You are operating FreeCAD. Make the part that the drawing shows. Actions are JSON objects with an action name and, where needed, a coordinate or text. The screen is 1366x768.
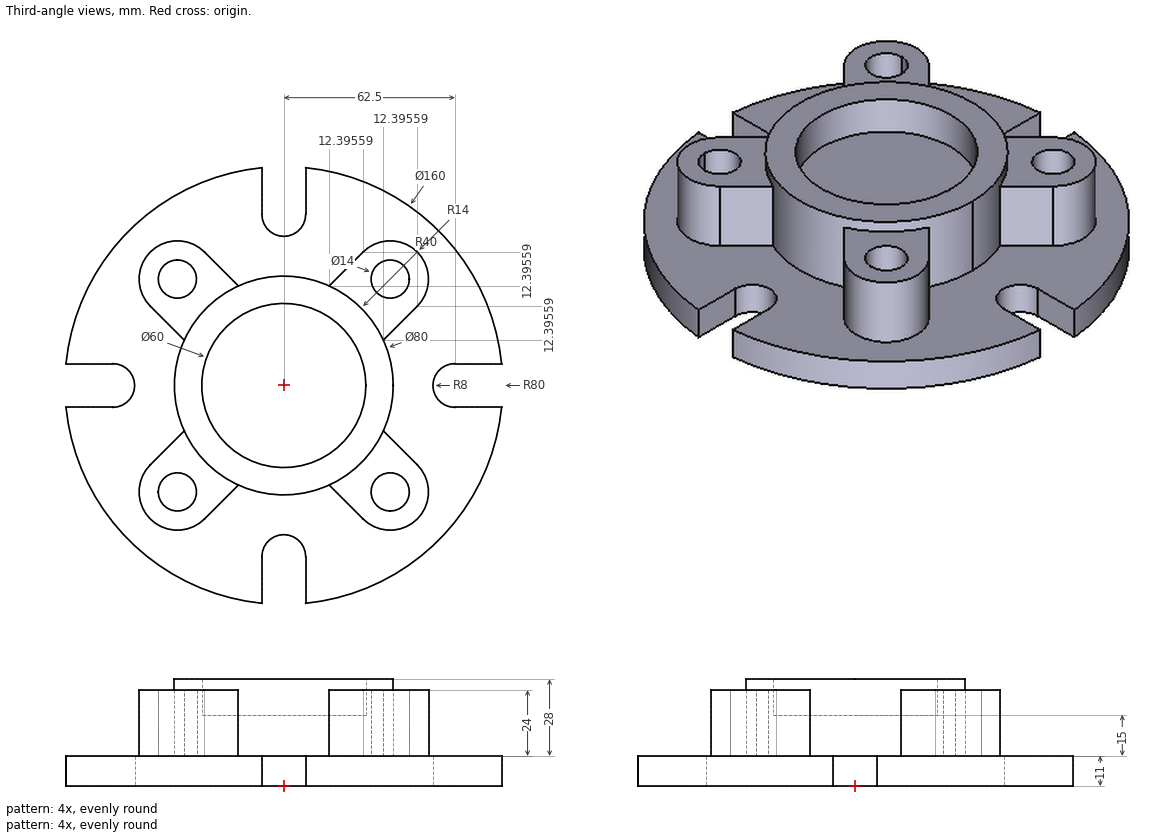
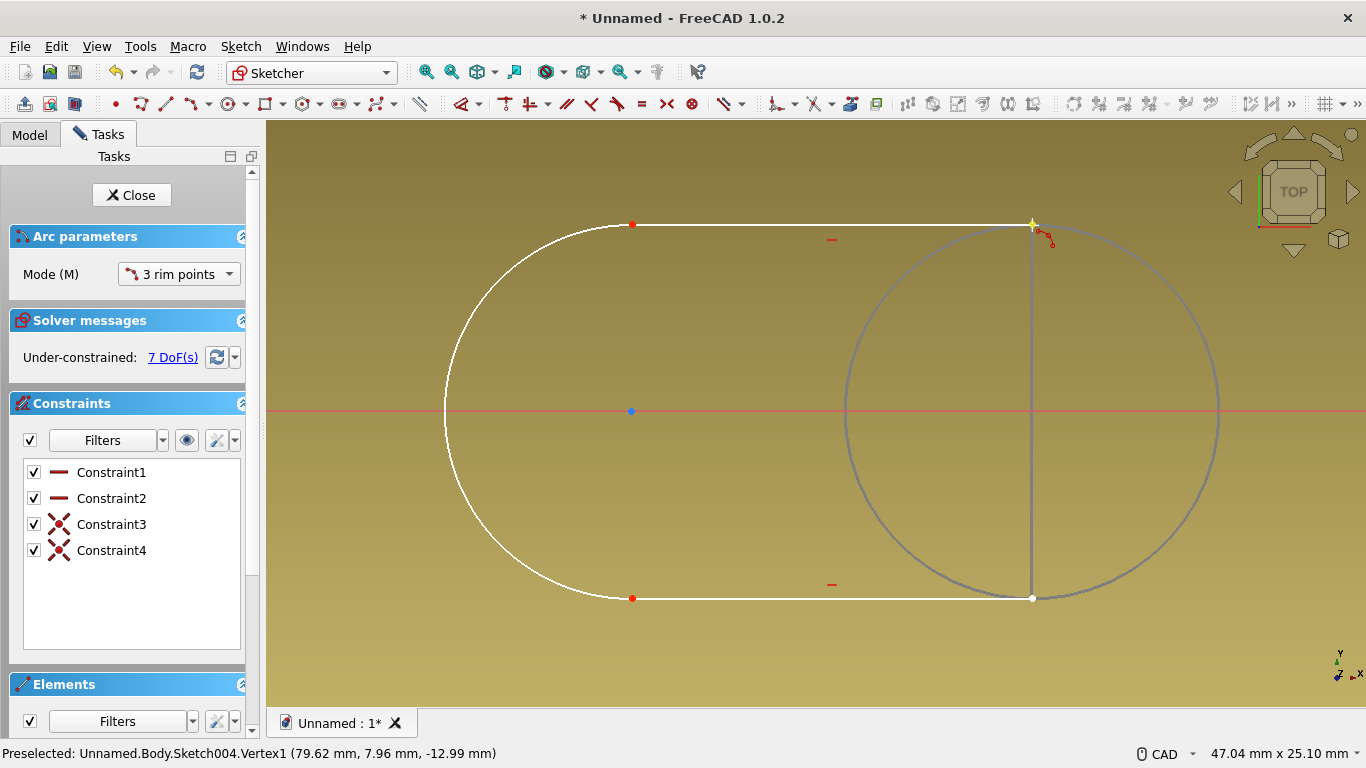
{"action": "scroll", "coordinate": [1041, 449], "scroll_direction": "up", "scroll_amount": 3}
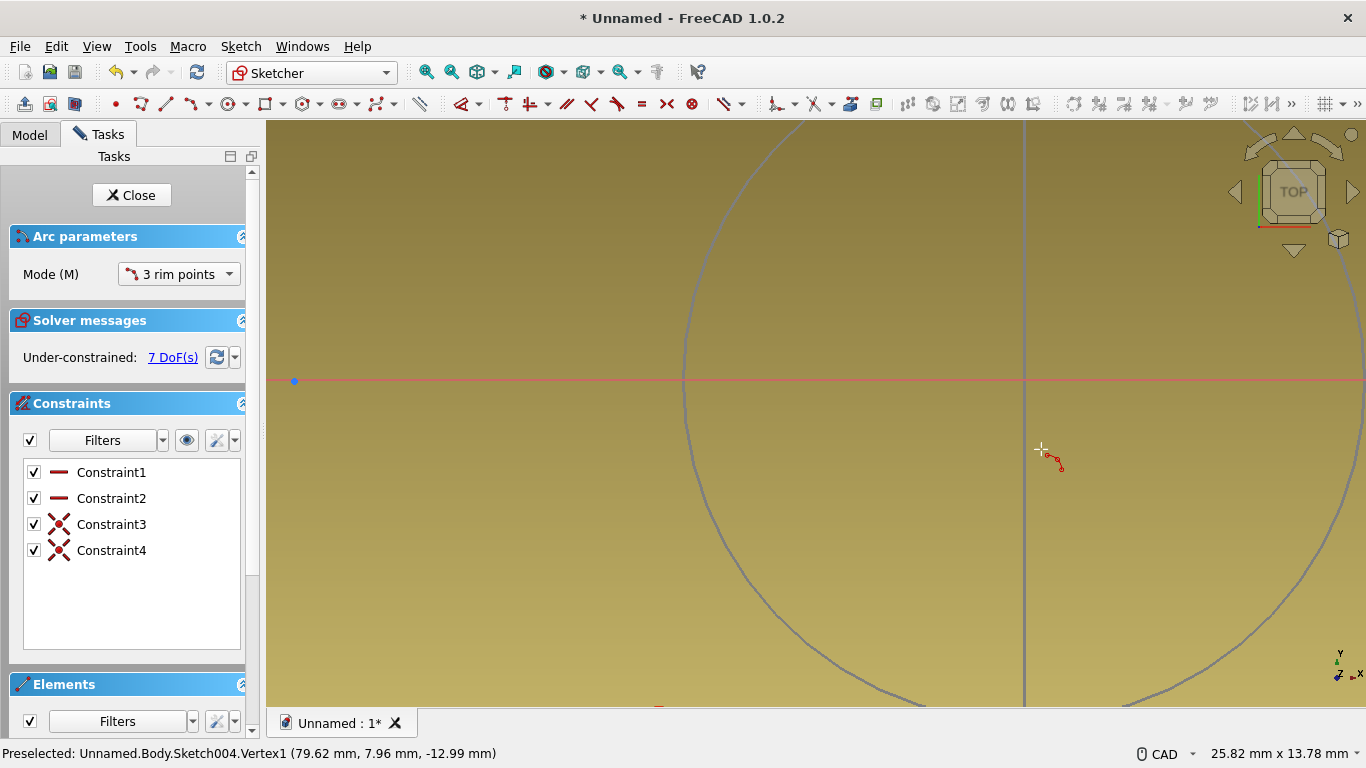
{"action": "left_click", "coordinate": [1040, 448]}
{"action": "key", "text": "Escape"}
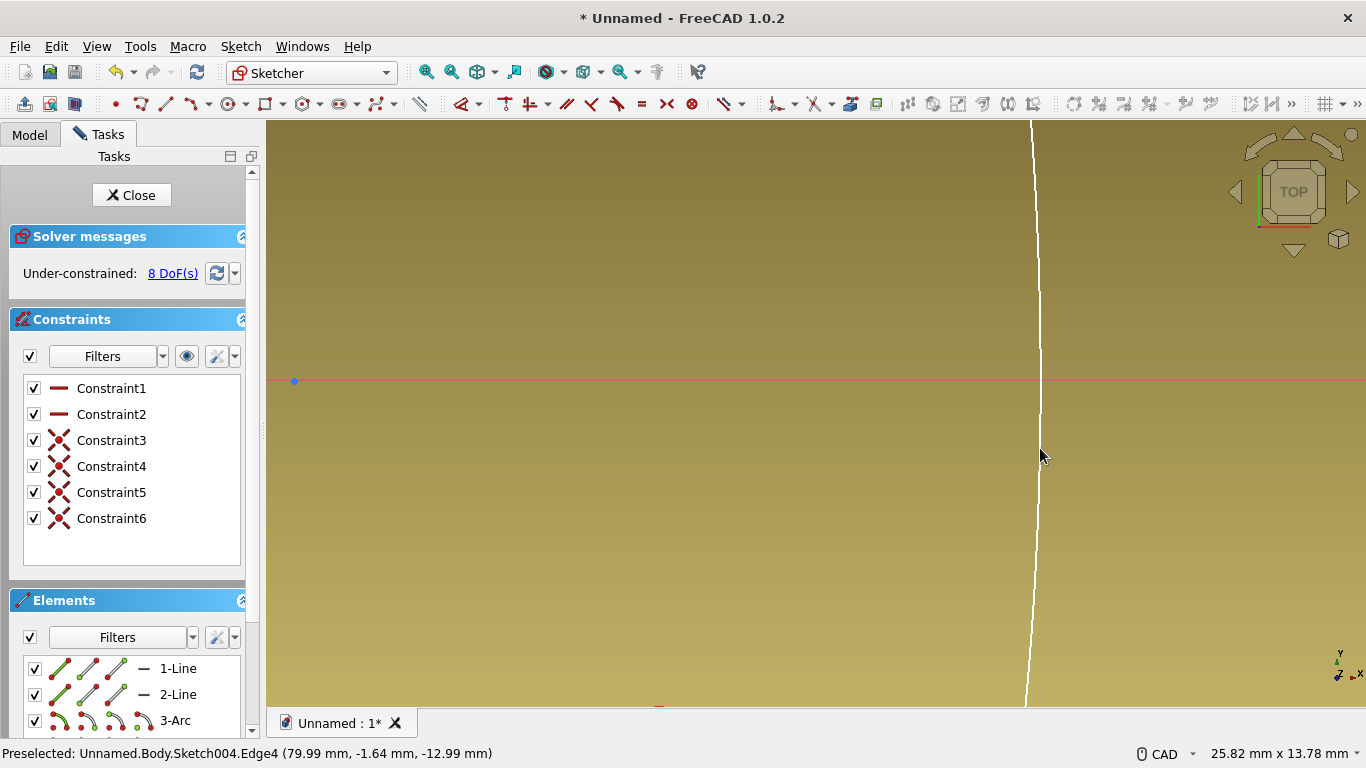
{"action": "scroll", "coordinate": [1052, 455], "scroll_direction": "down", "scroll_amount": 3}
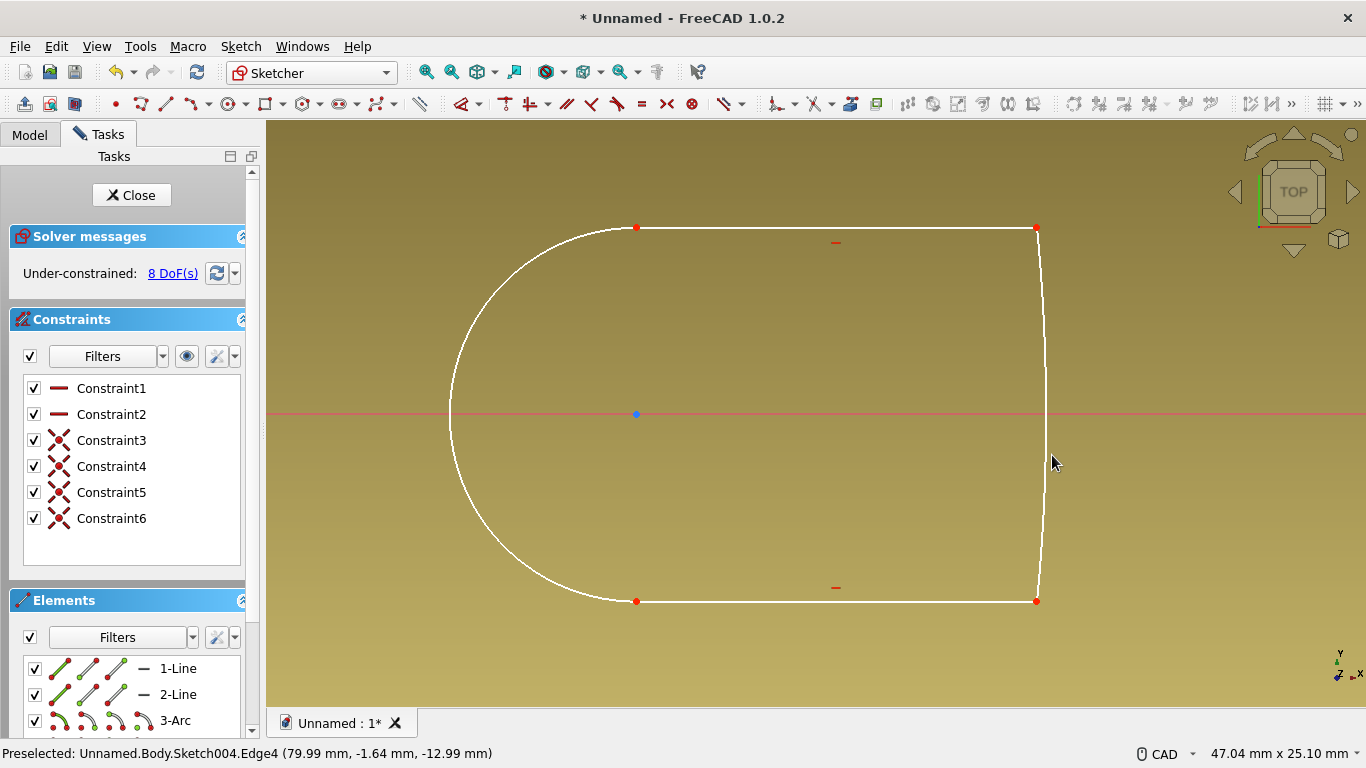
{"action": "left_click", "coordinate": [917, 228]}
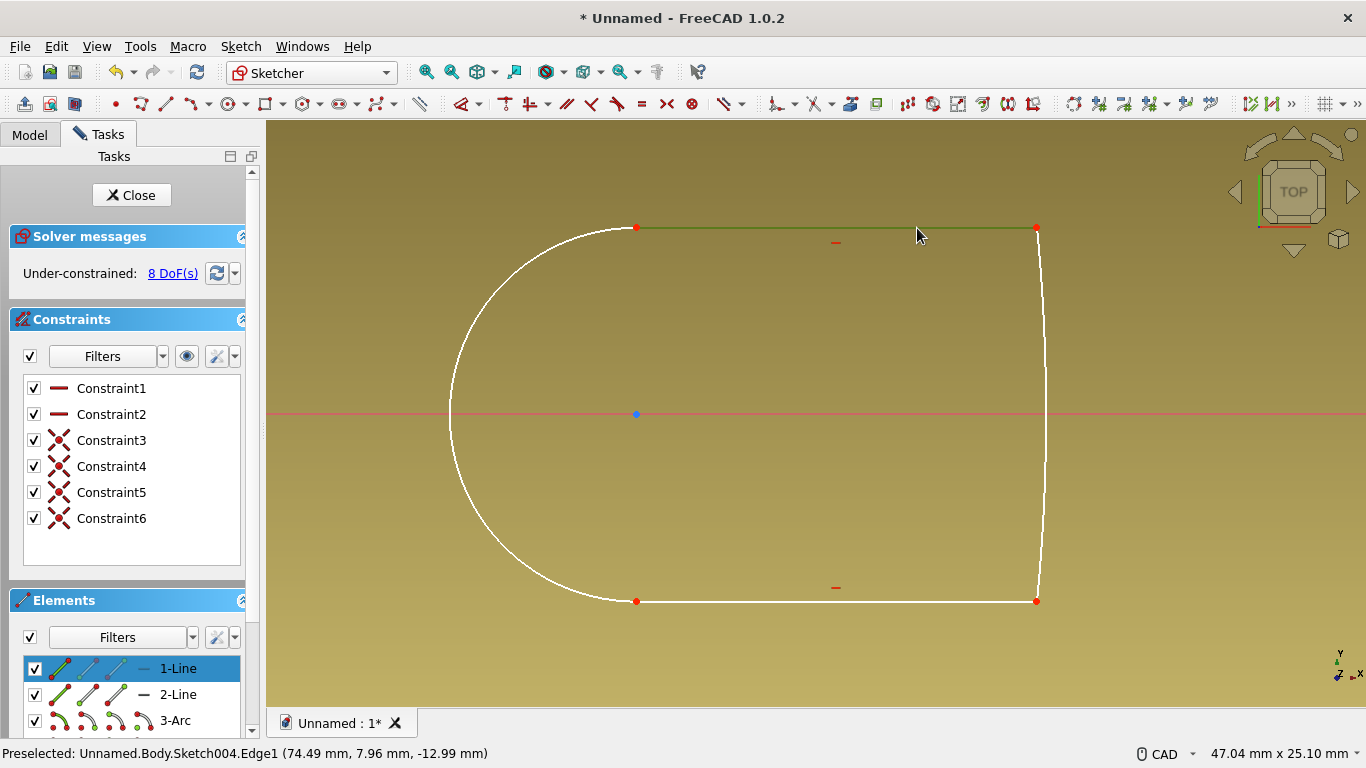
{"action": "left_click", "coordinate": [486, 305]}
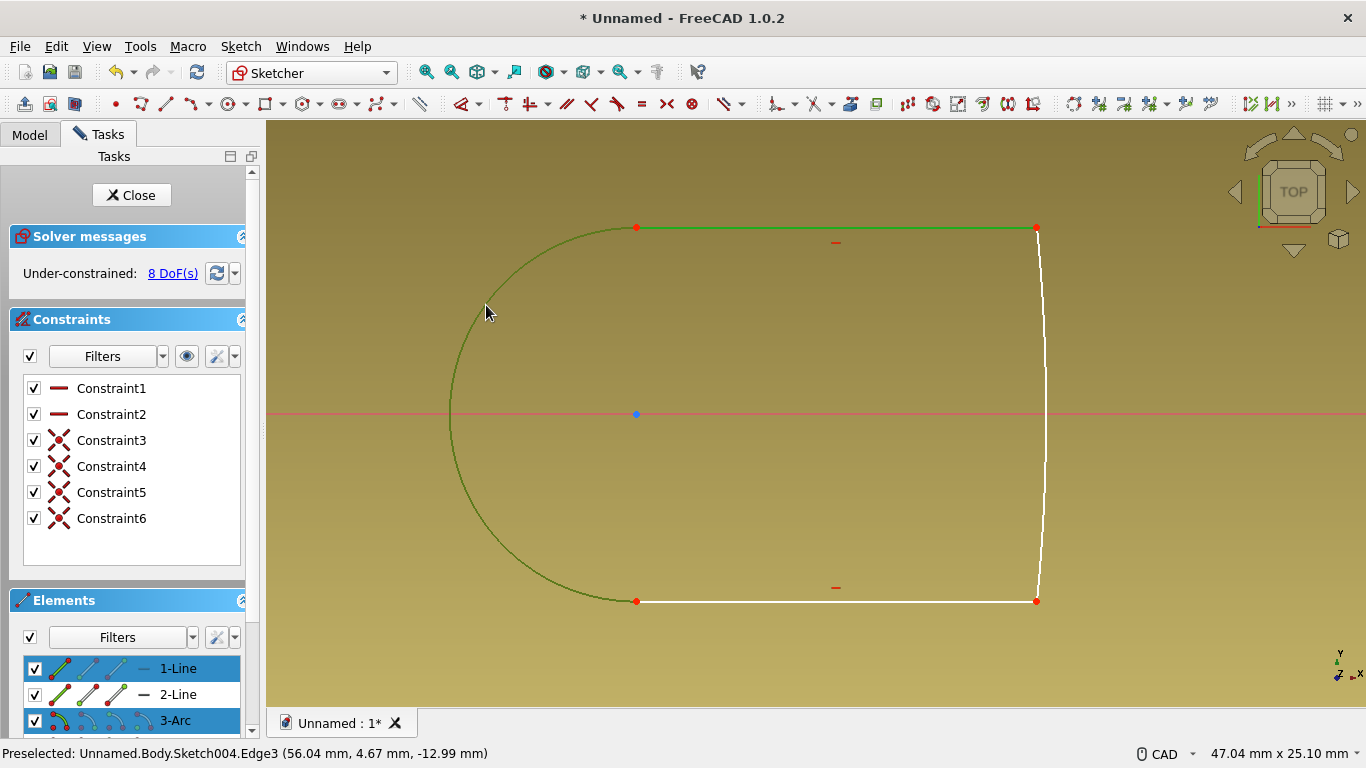
{"action": "key", "text": "t"}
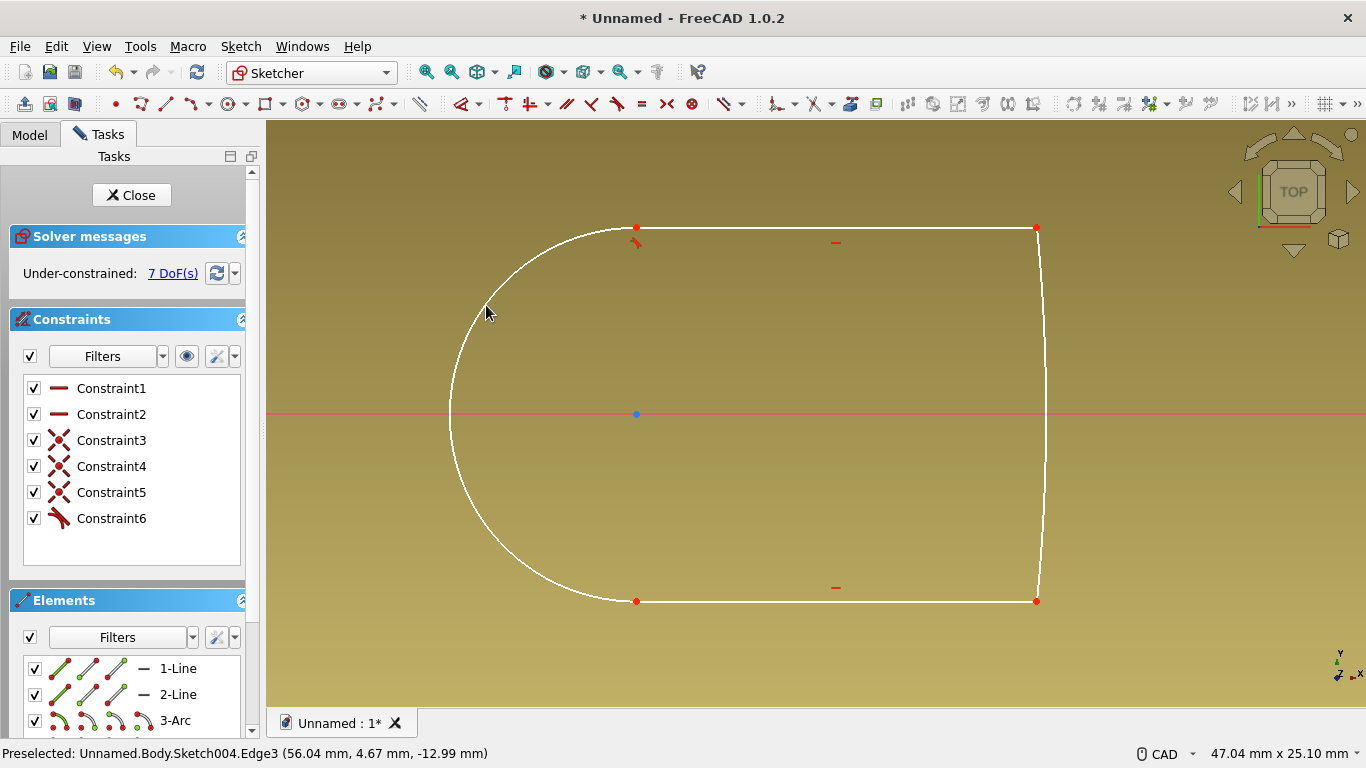
{"action": "left_click", "coordinate": [757, 602]}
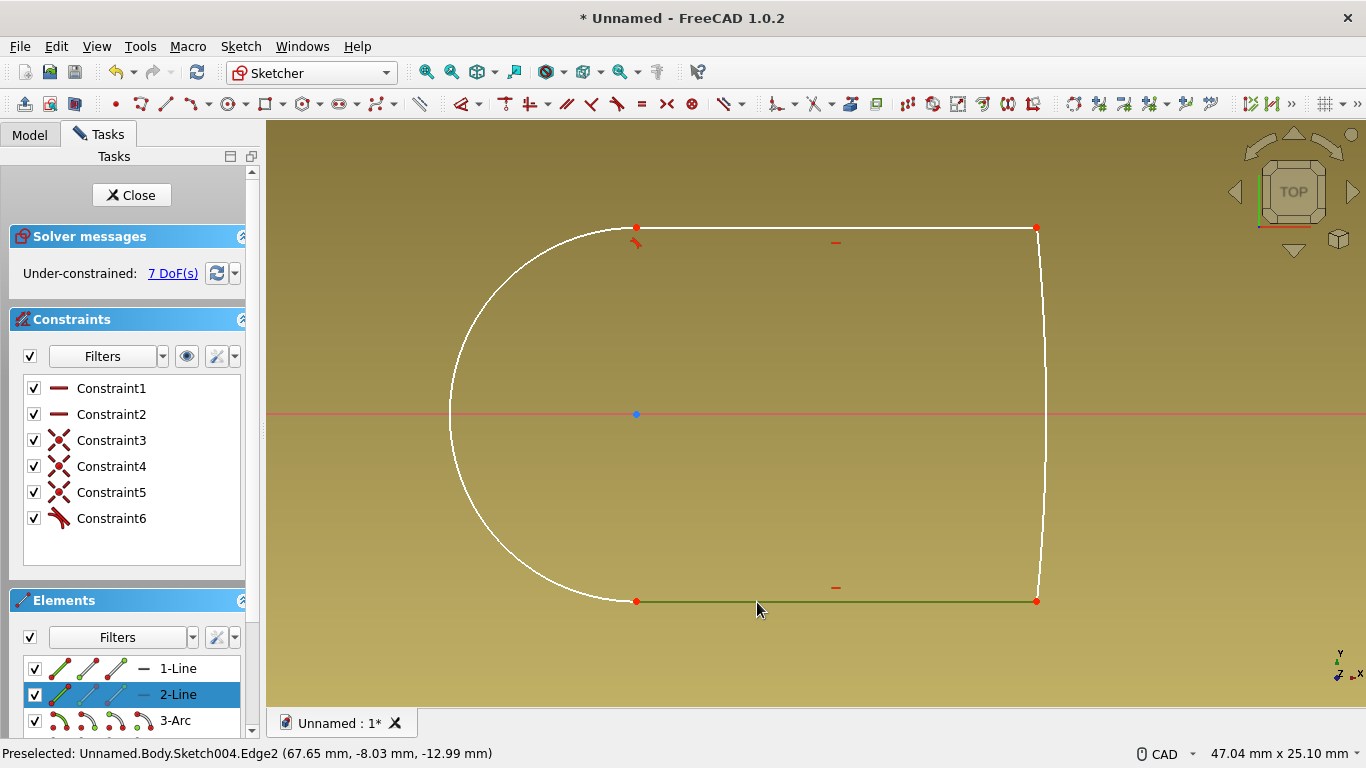
{"action": "left_click", "coordinate": [485, 305]}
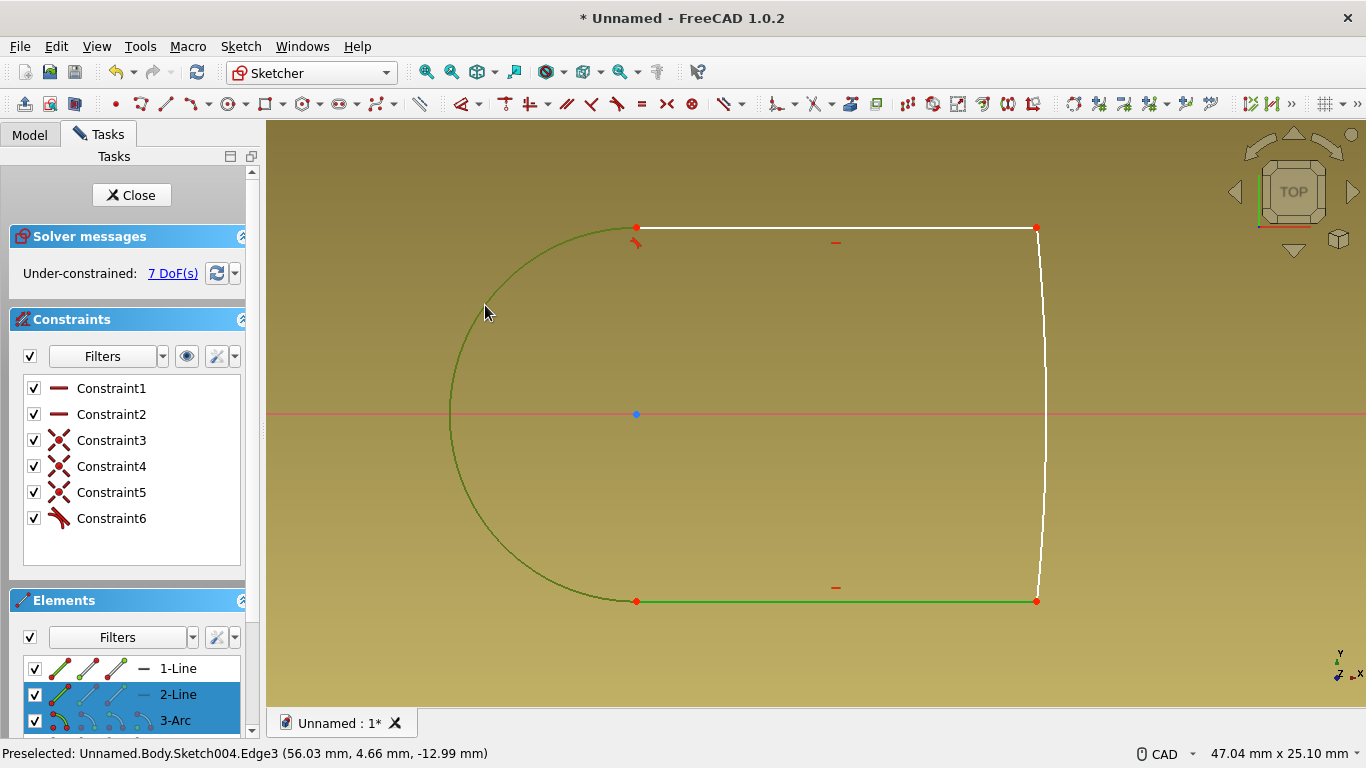
{"action": "key", "text": "t"}